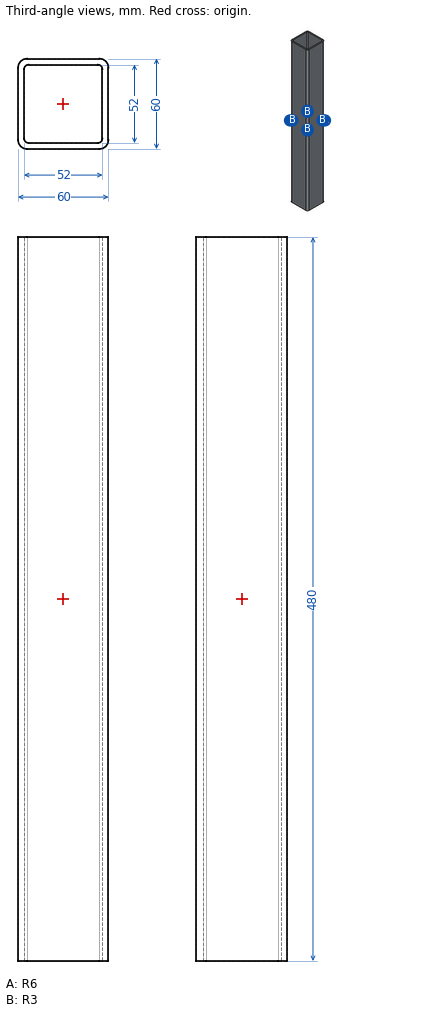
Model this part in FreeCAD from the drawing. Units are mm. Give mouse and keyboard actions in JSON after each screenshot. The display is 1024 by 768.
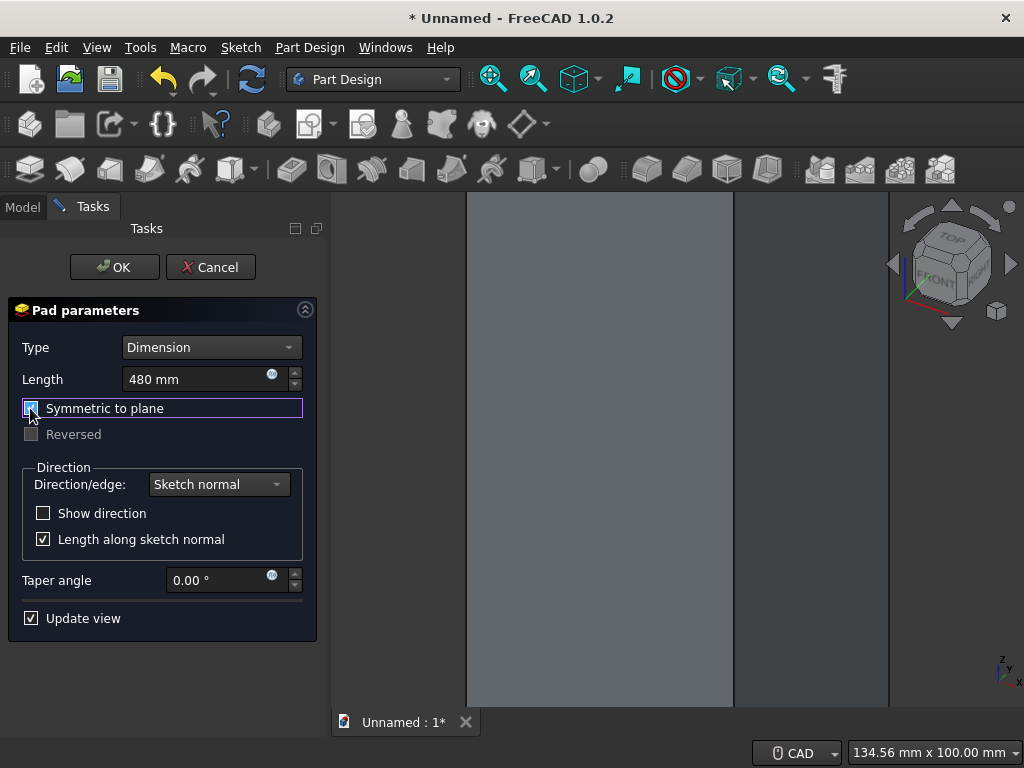
{"action": "left_click", "coordinate": [115, 267]}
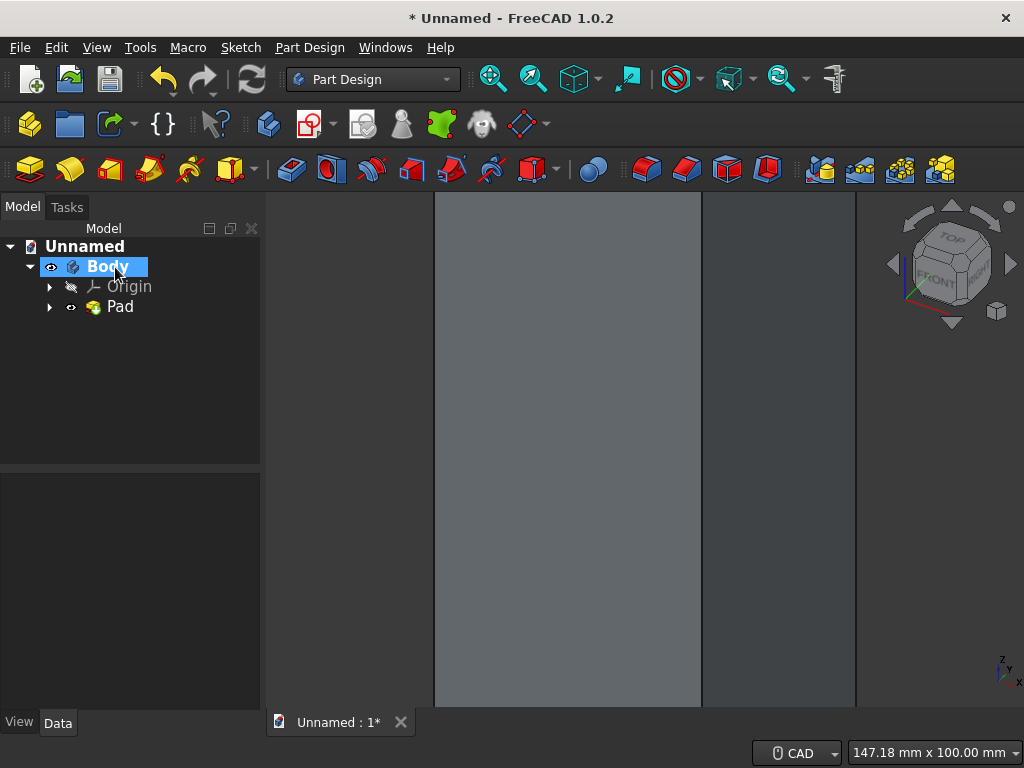
{"action": "key", "text": "v f"}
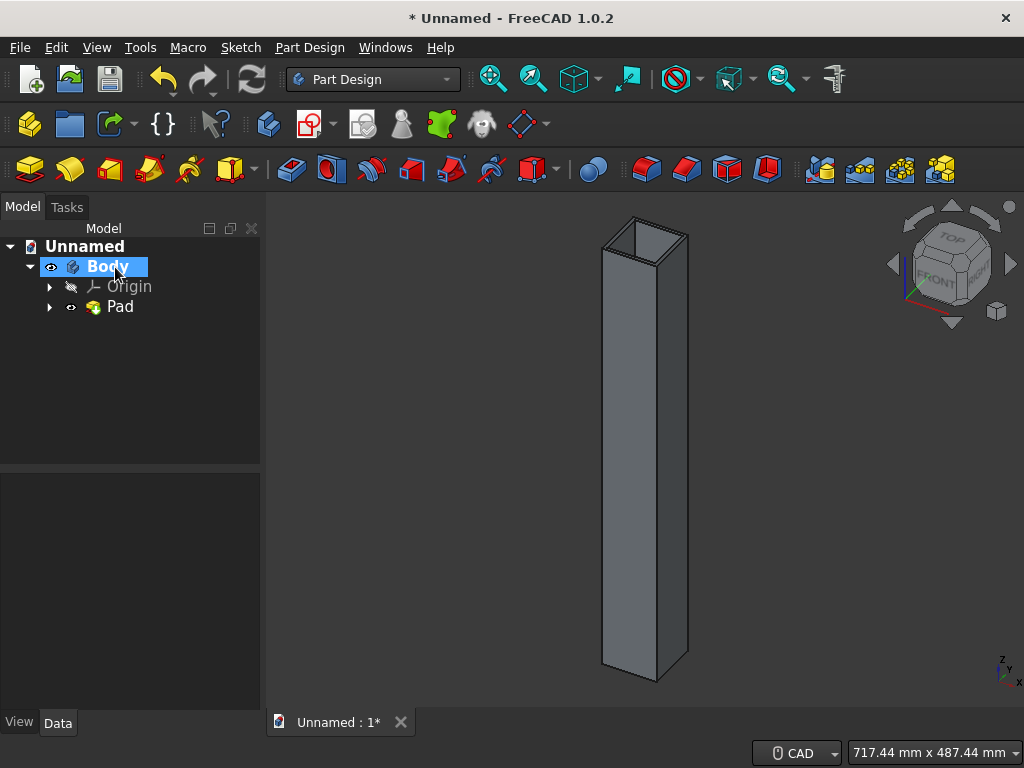
{"action": "left_click", "coordinate": [657, 473]}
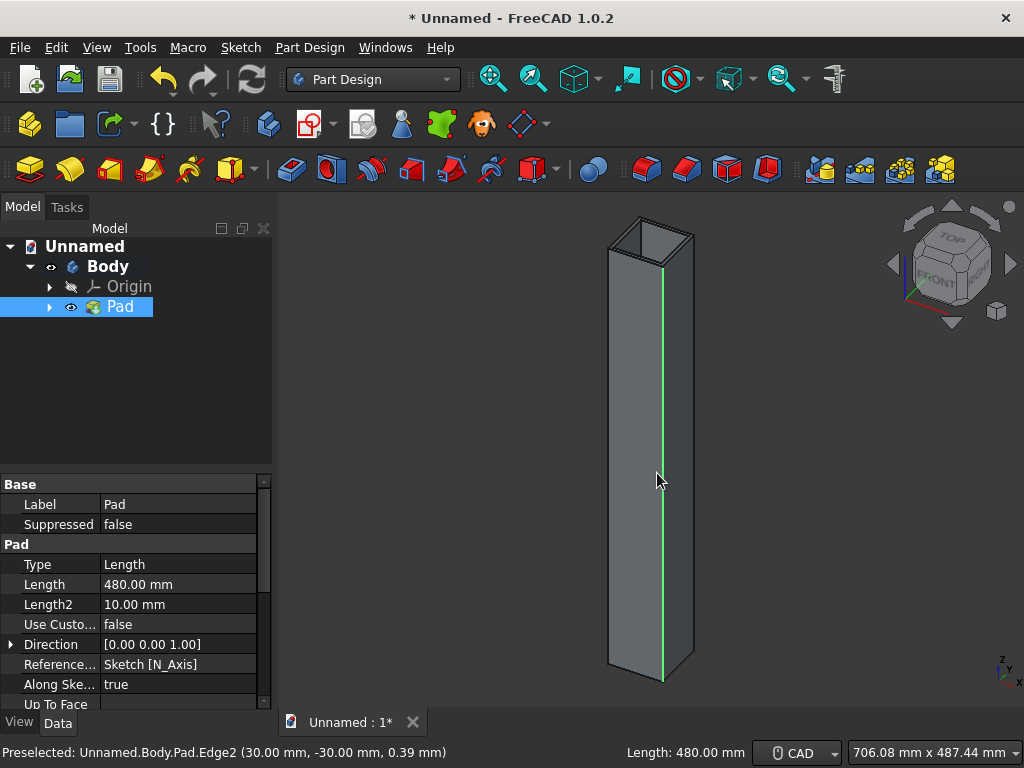
{"action": "key", "text": "0"}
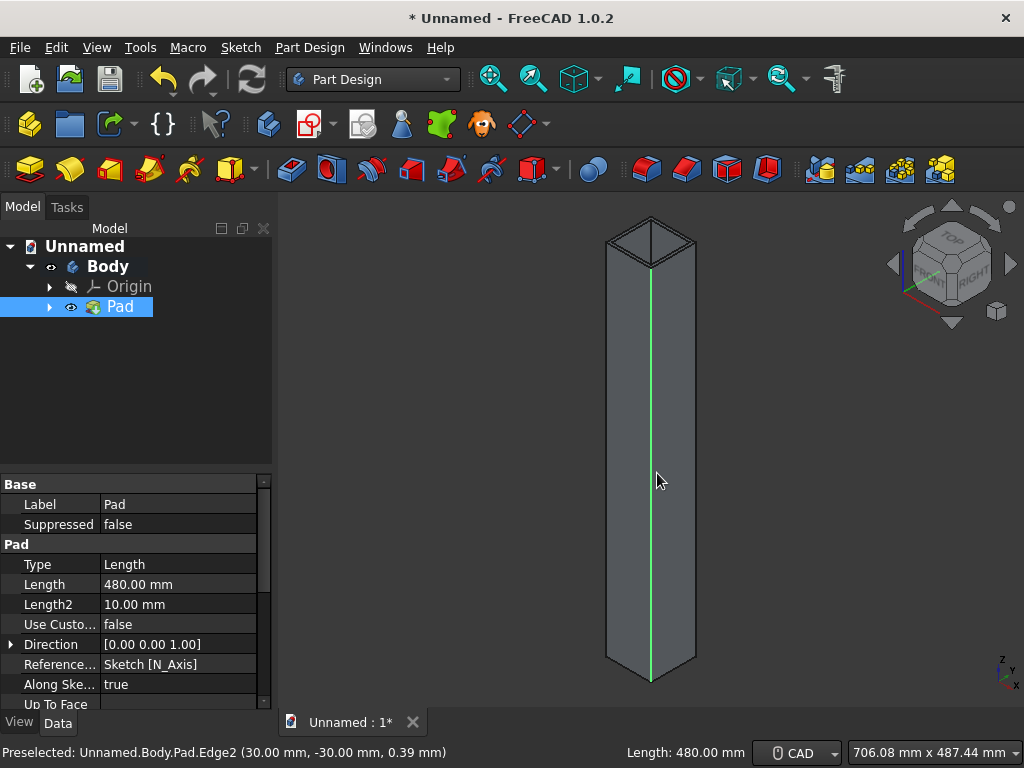
{"action": "key", "text": "2"}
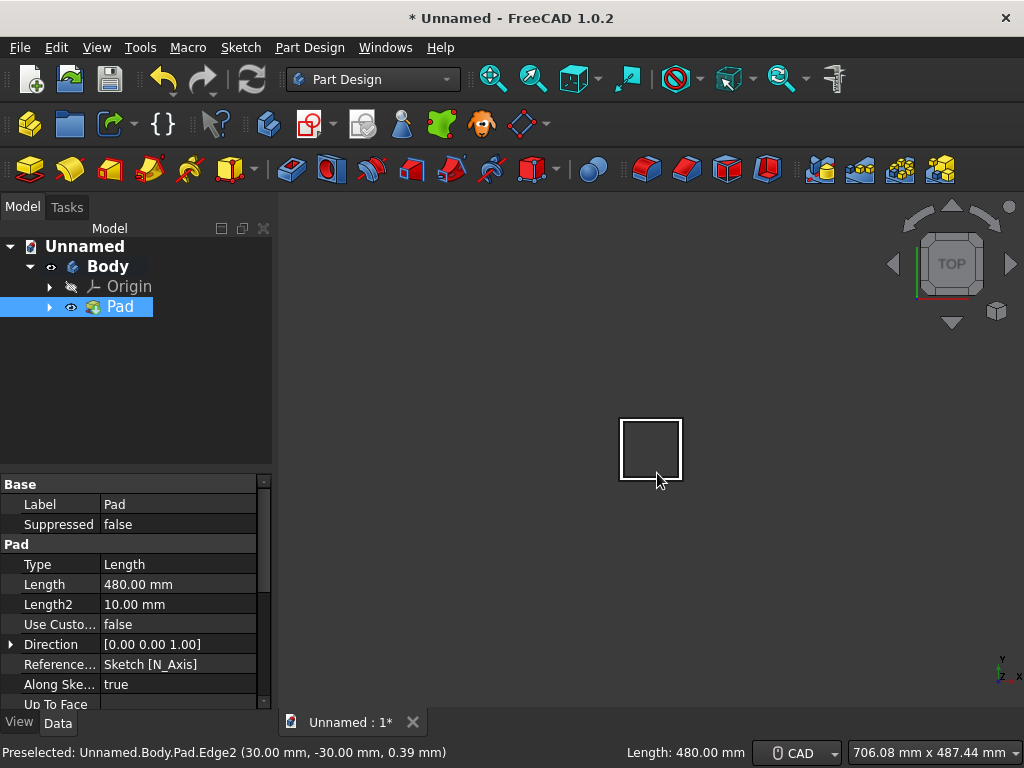
{"action": "left_click", "coordinate": [494, 80]}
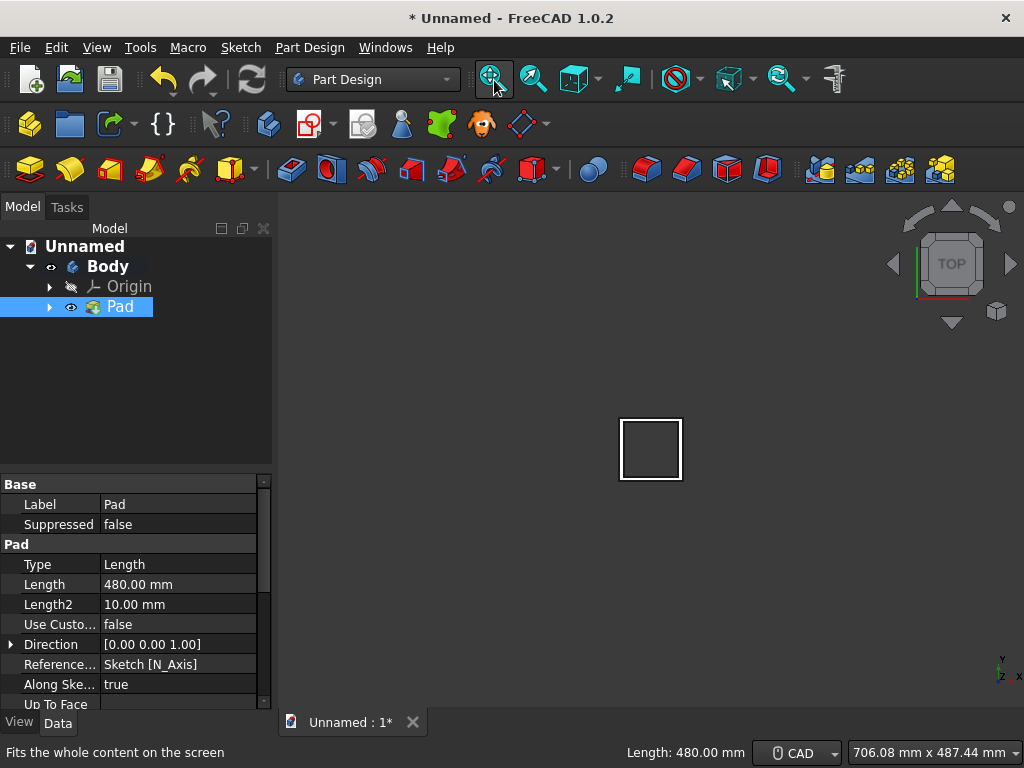
{"action": "key", "text": "1"}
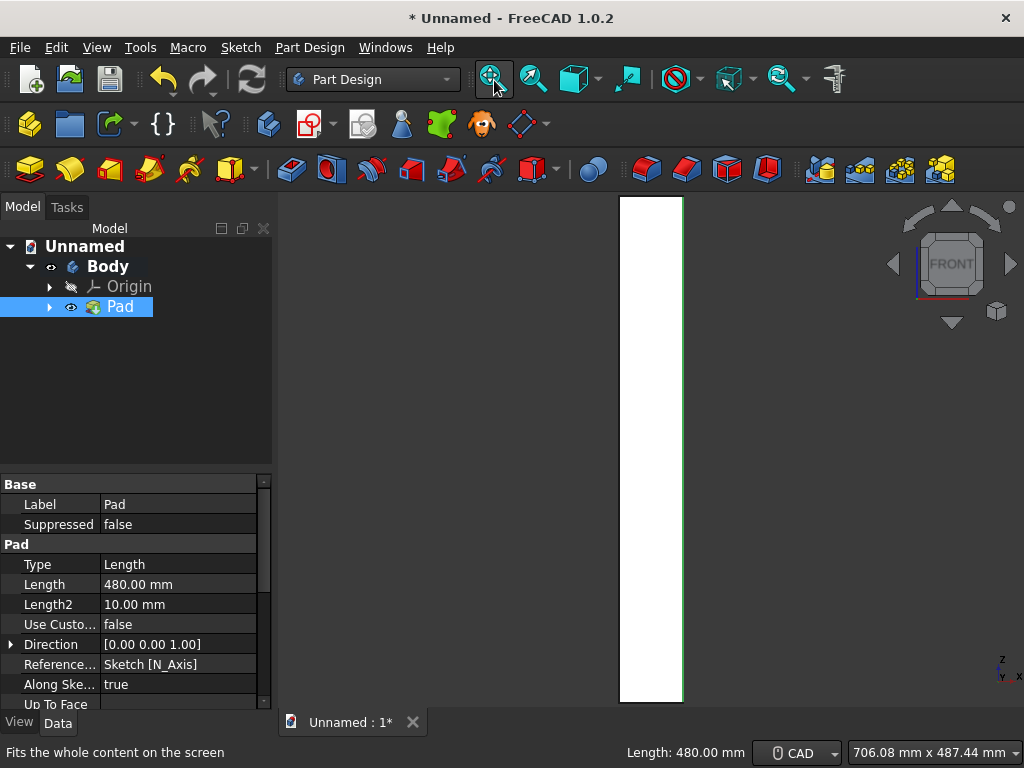
{"action": "left_click", "coordinate": [619, 449], "text": "ctrl"}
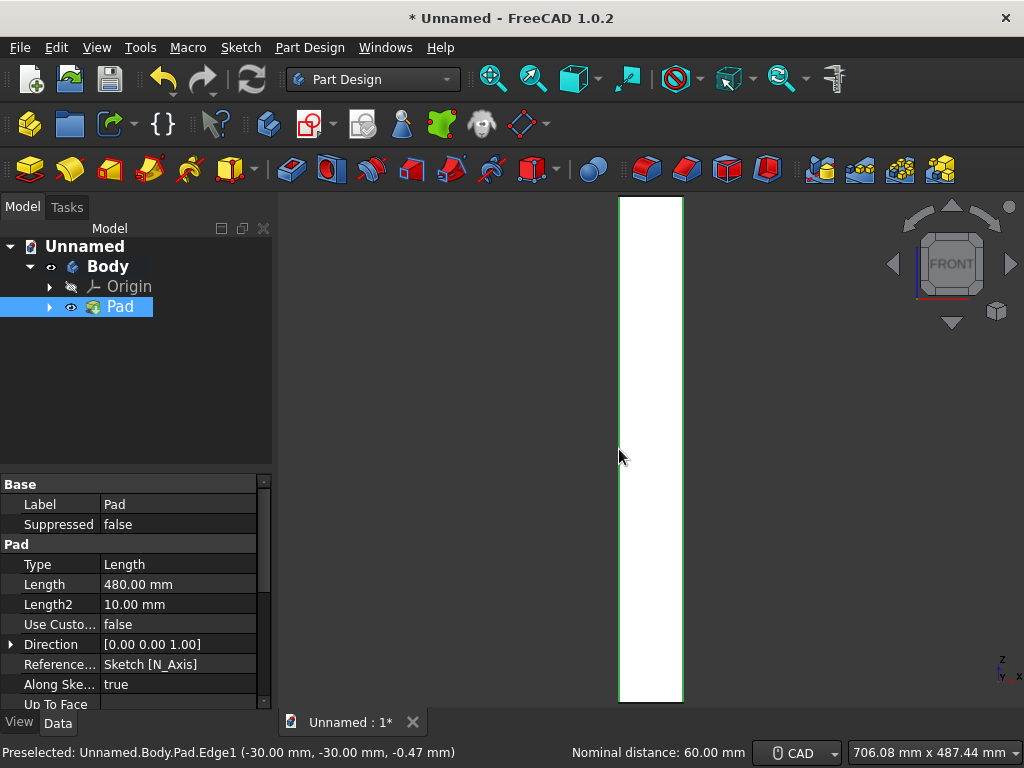
{"action": "key", "text": "3"}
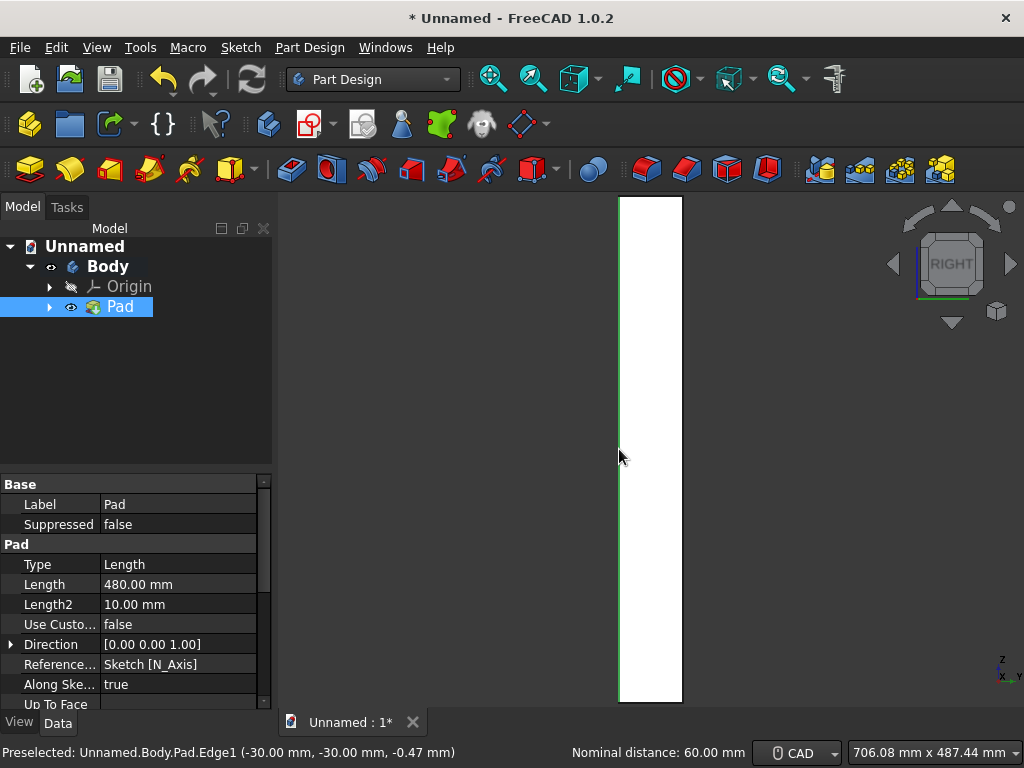
{"action": "left_click", "coordinate": [683, 448], "text": "ctrl"}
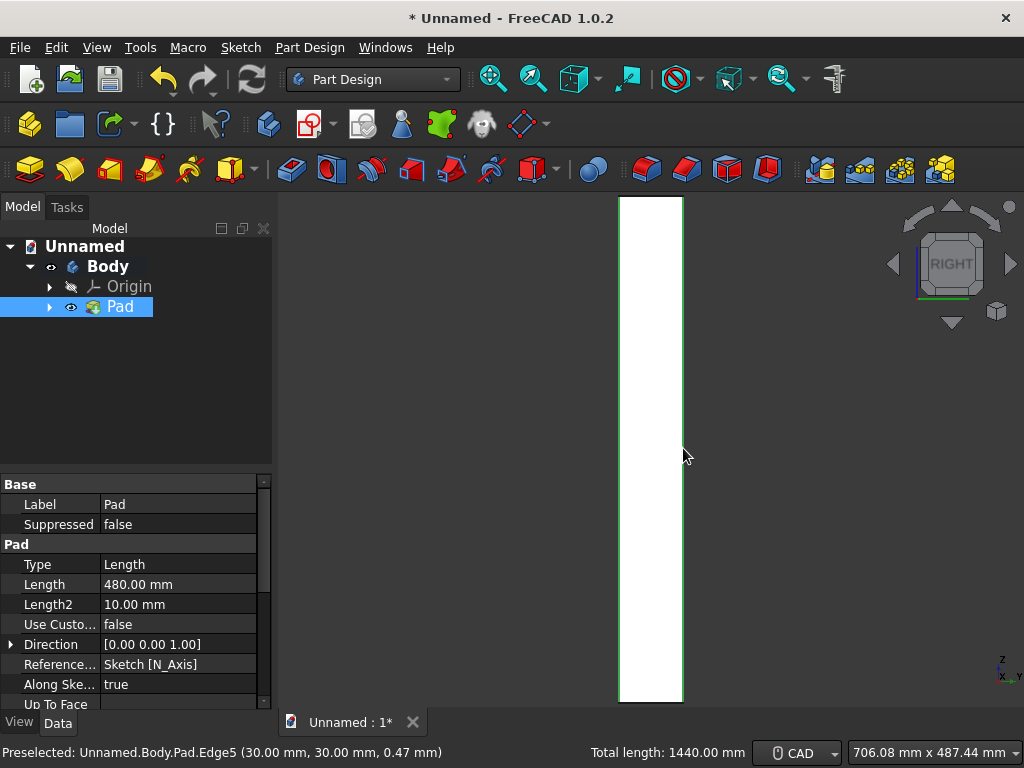
{"action": "key", "text": "5"}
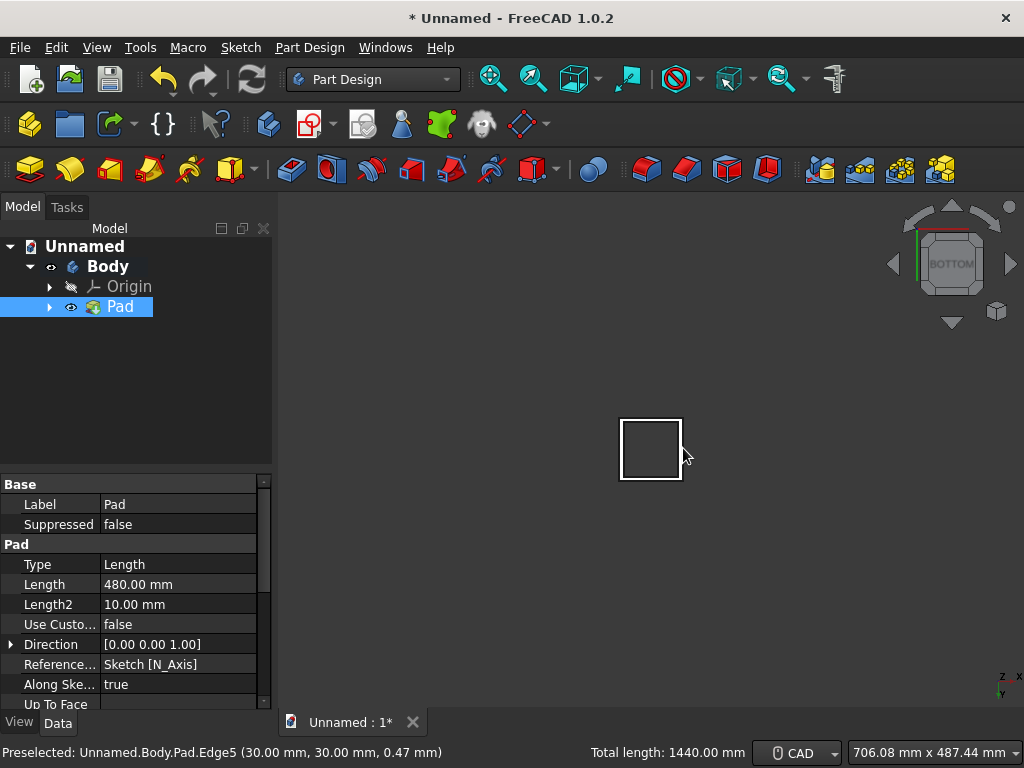
{"action": "left_click", "coordinate": [494, 80]}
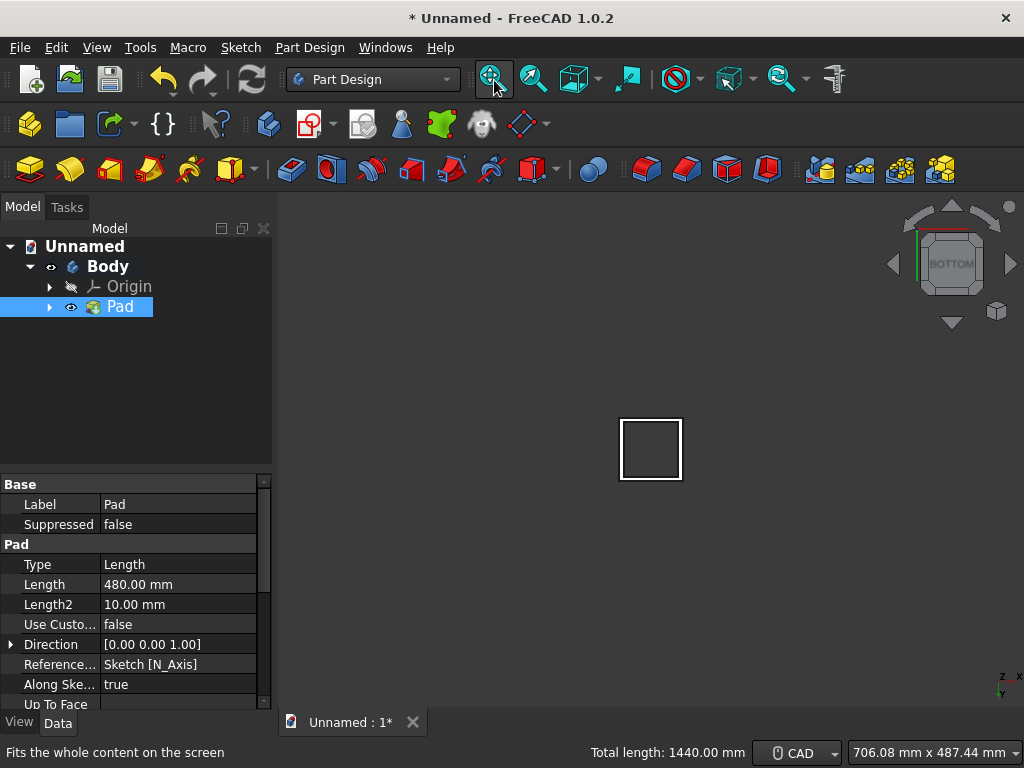
{"action": "key", "text": "4"}